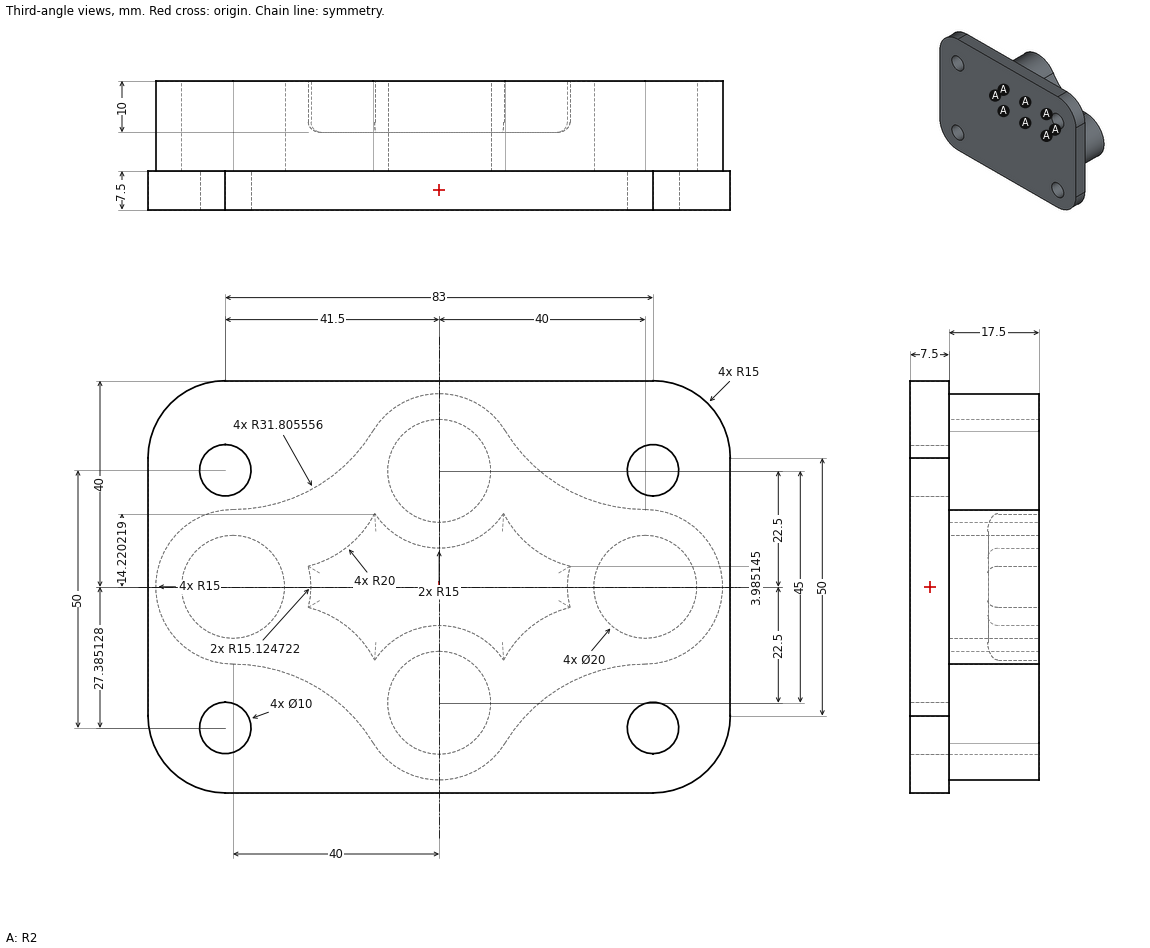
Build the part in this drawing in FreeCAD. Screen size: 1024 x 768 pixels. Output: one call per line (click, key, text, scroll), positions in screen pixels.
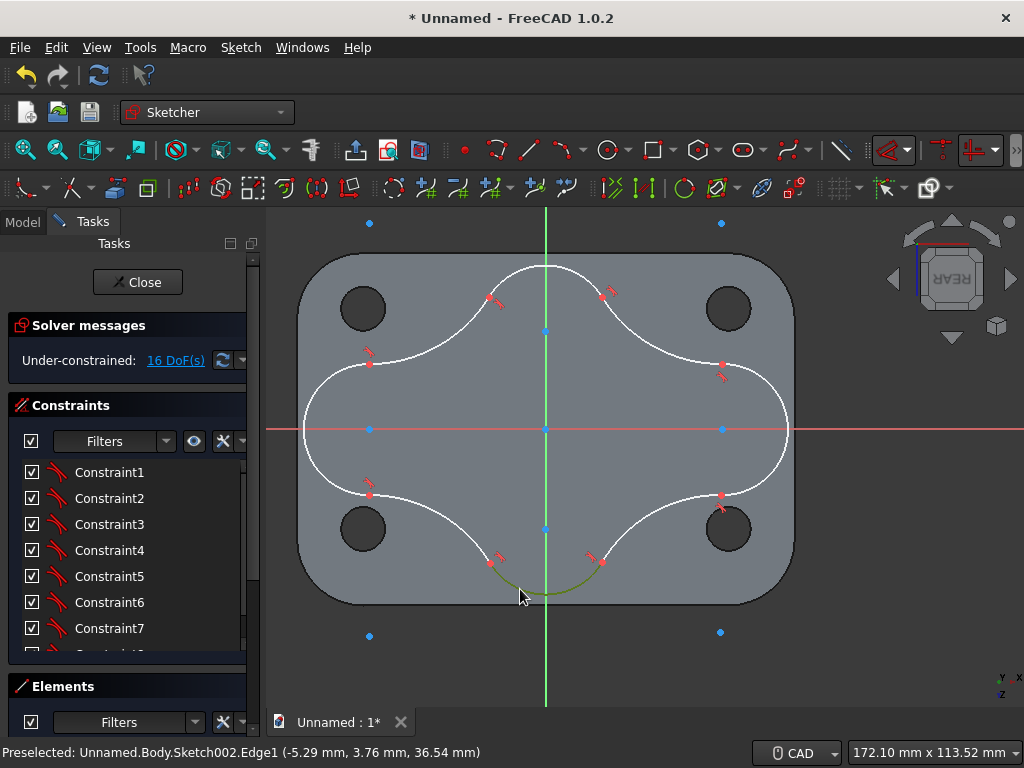
click(775, 468)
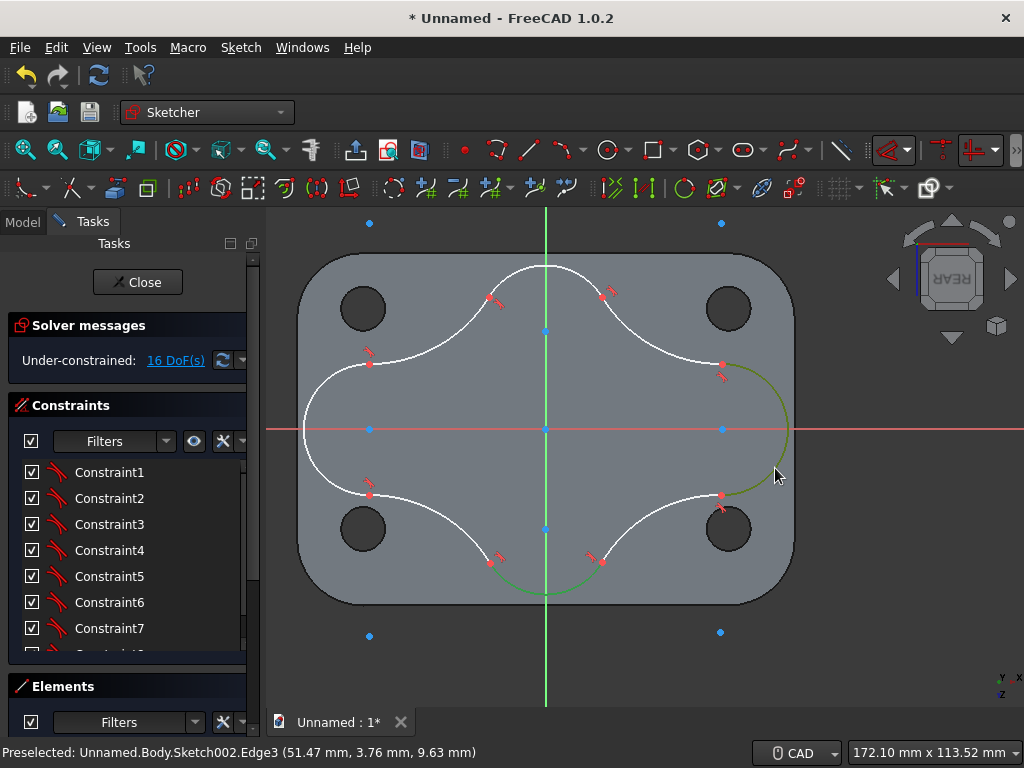
click(572, 271)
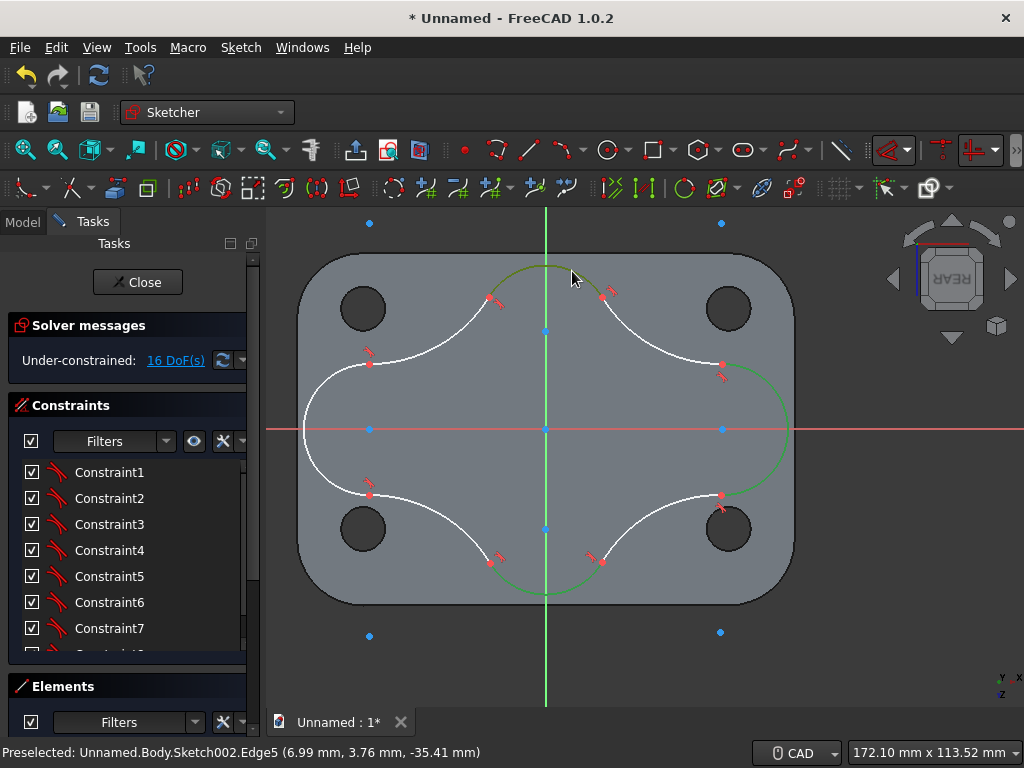
click(316, 391)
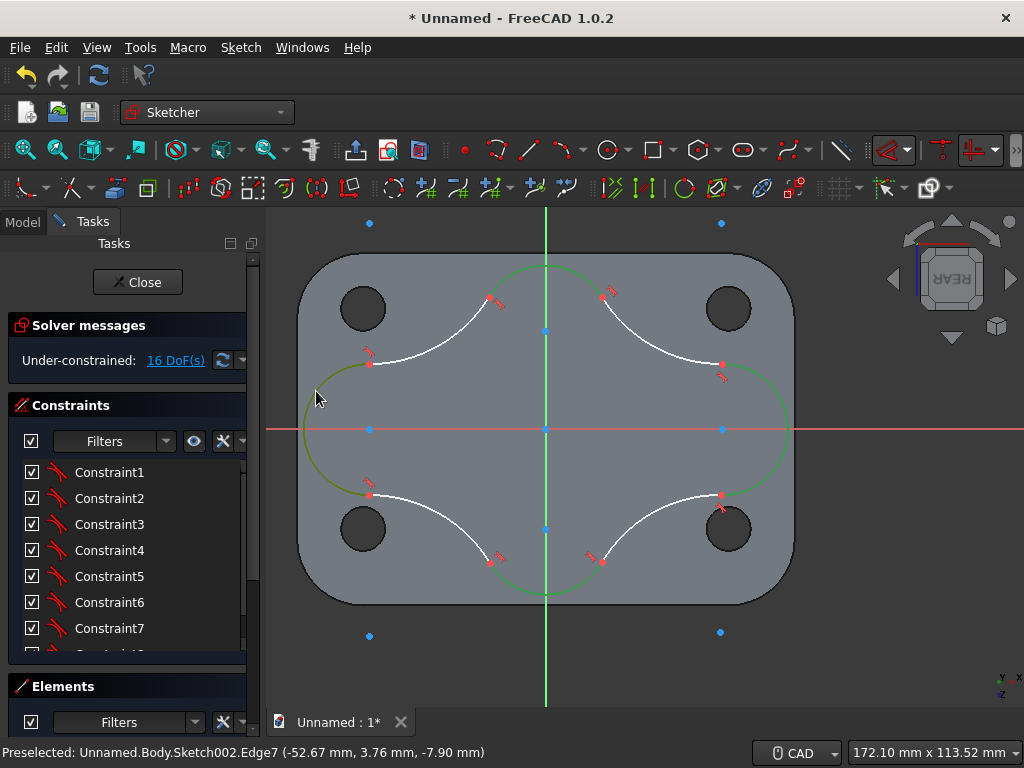
key(e)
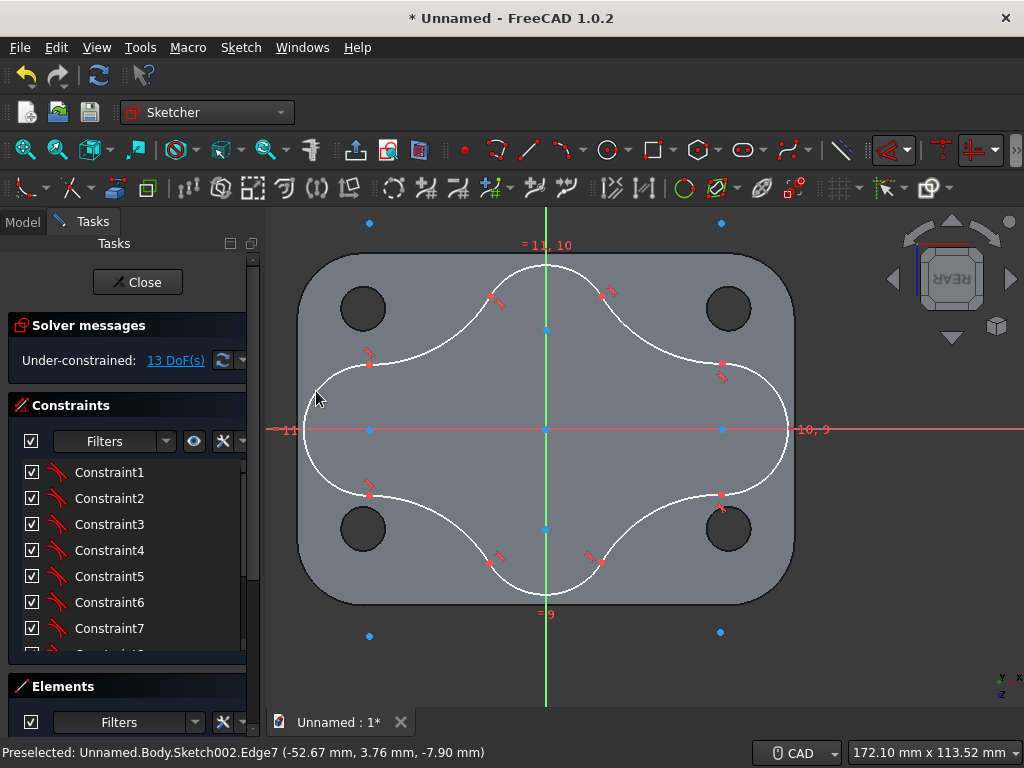
click(679, 501)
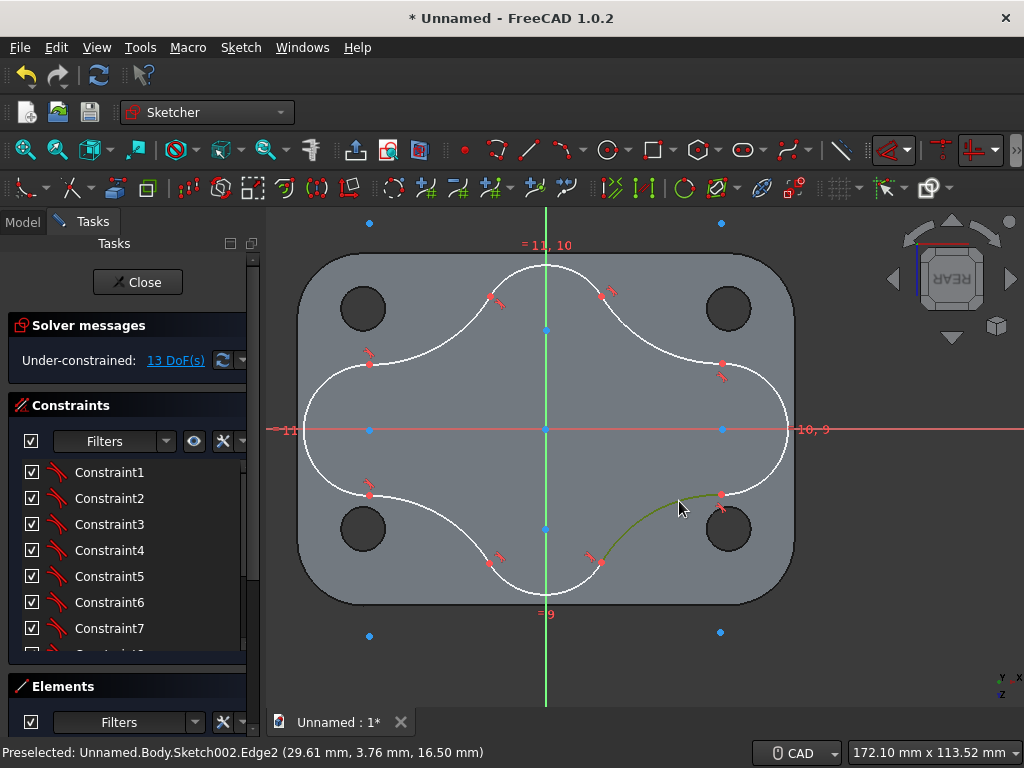
click(630, 329)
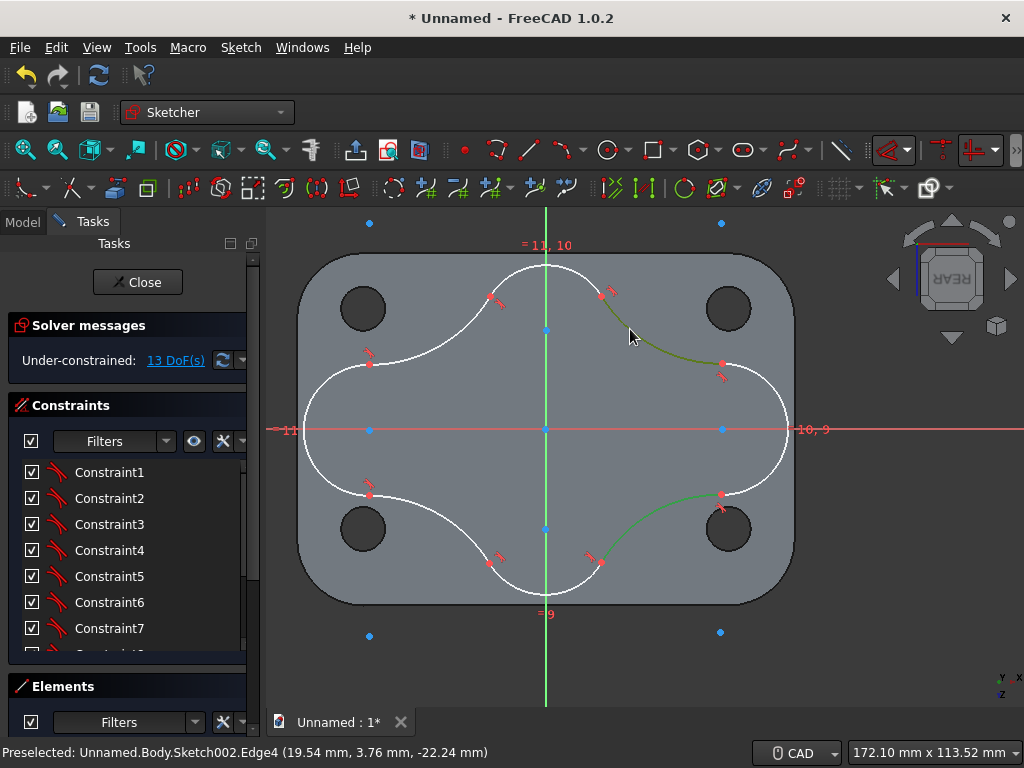
click(412, 358)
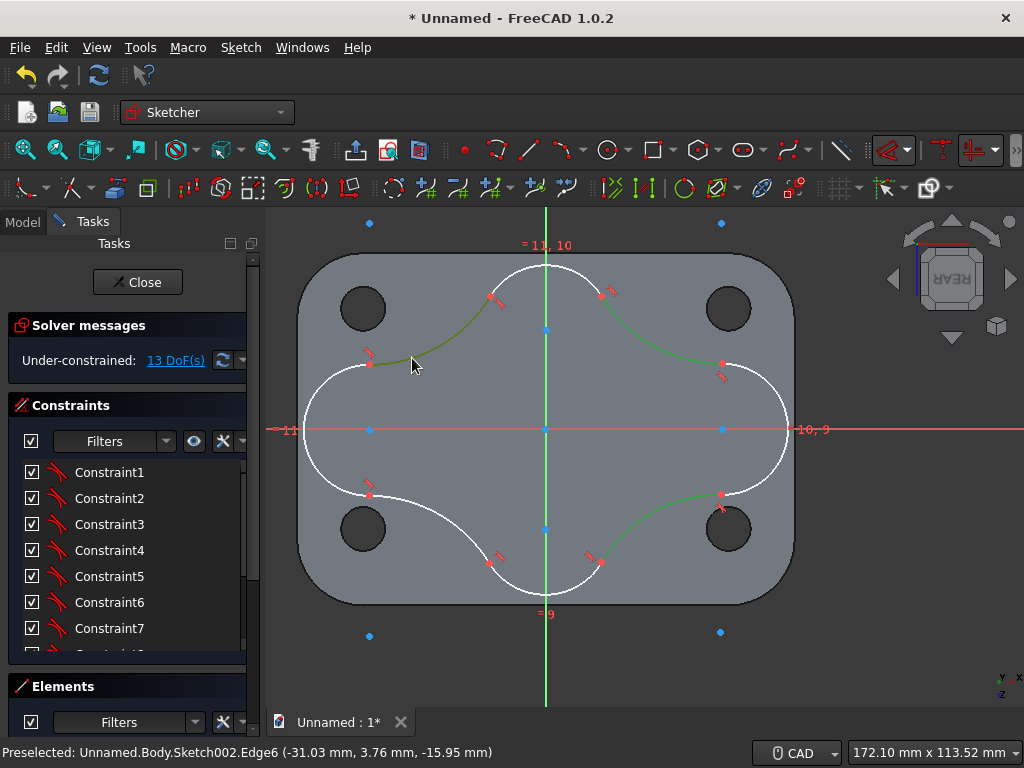
click(462, 530)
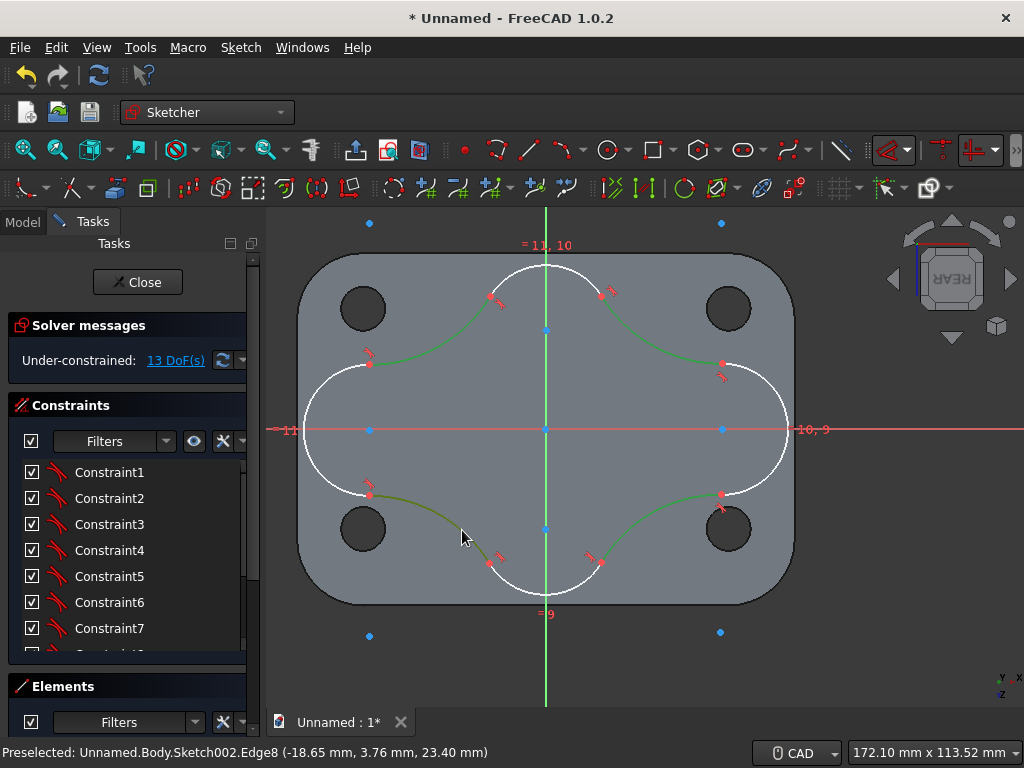
key(e)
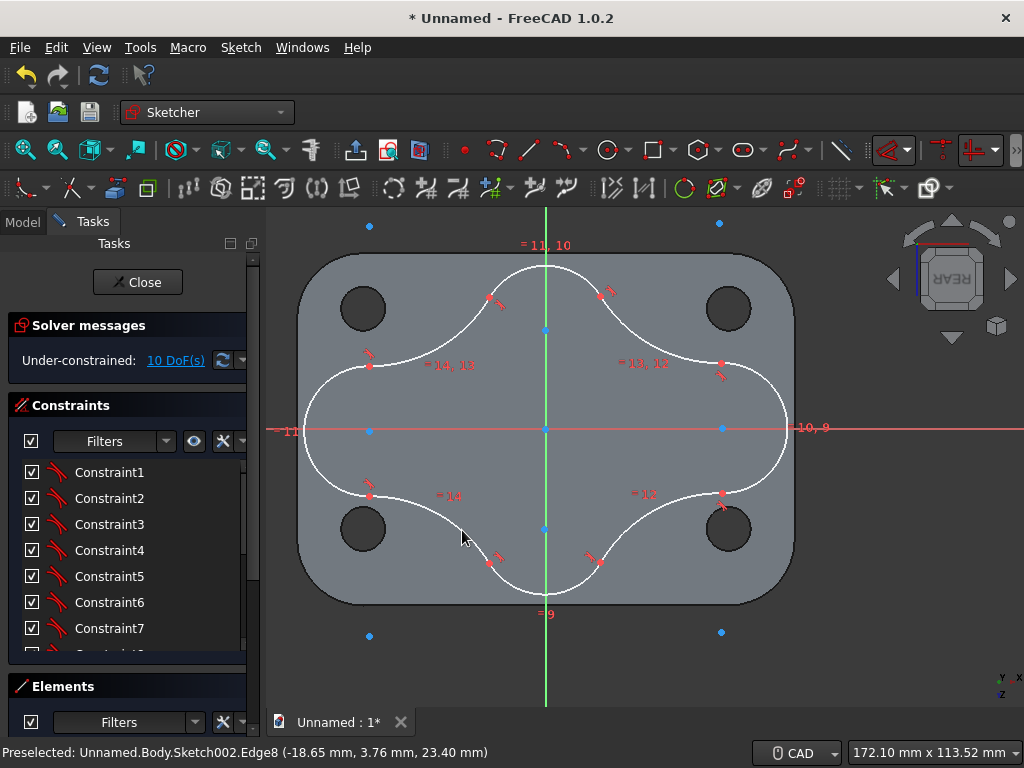
click(545, 530)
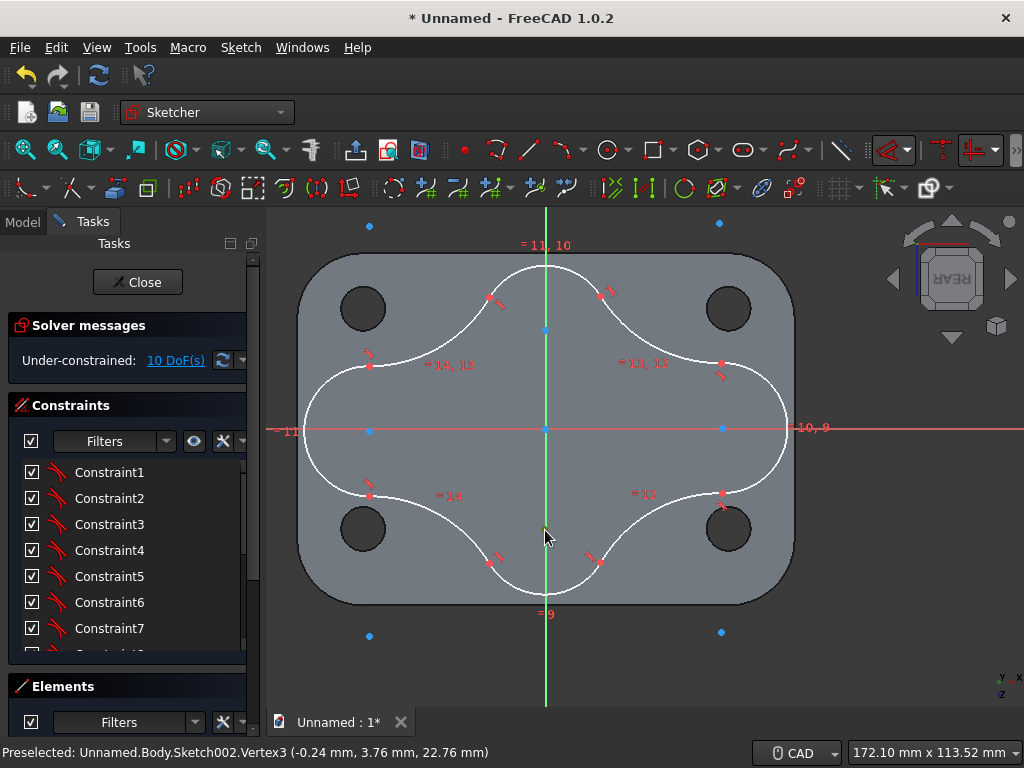
click(546, 647)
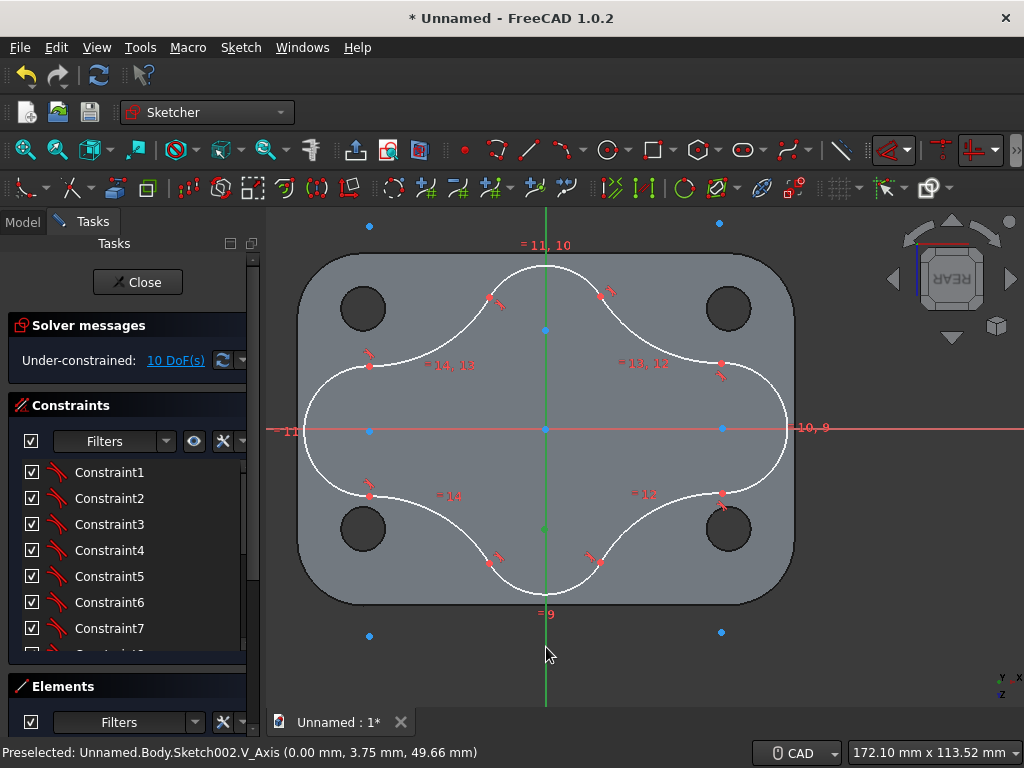
click(942, 150)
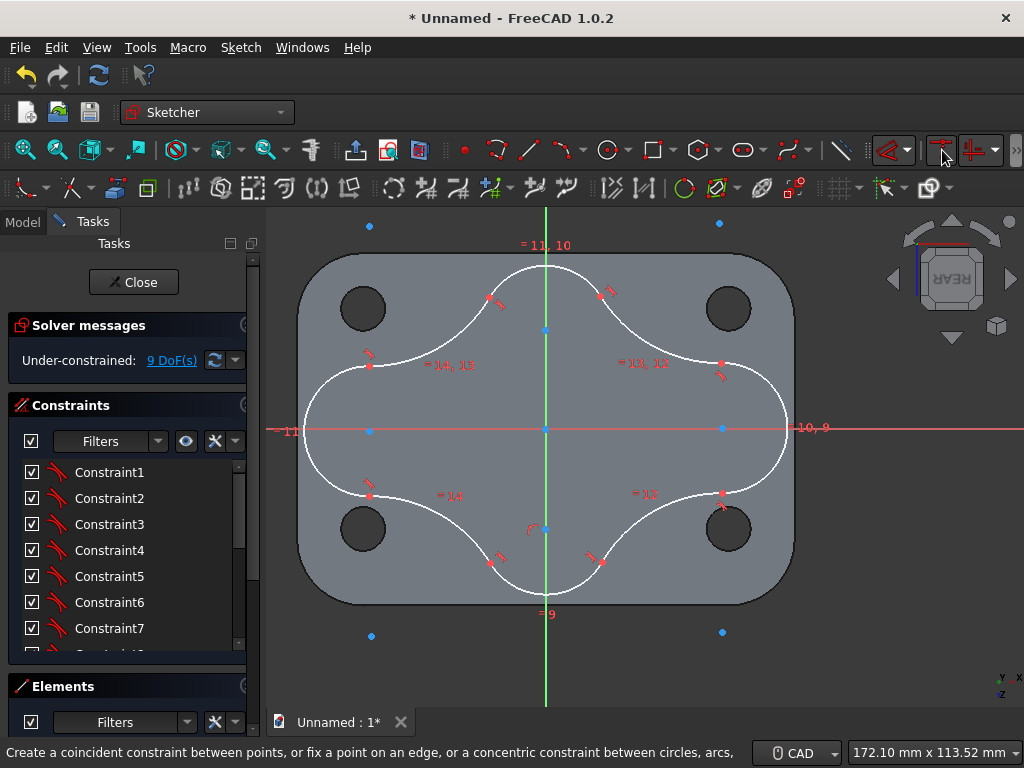
click(722, 428)